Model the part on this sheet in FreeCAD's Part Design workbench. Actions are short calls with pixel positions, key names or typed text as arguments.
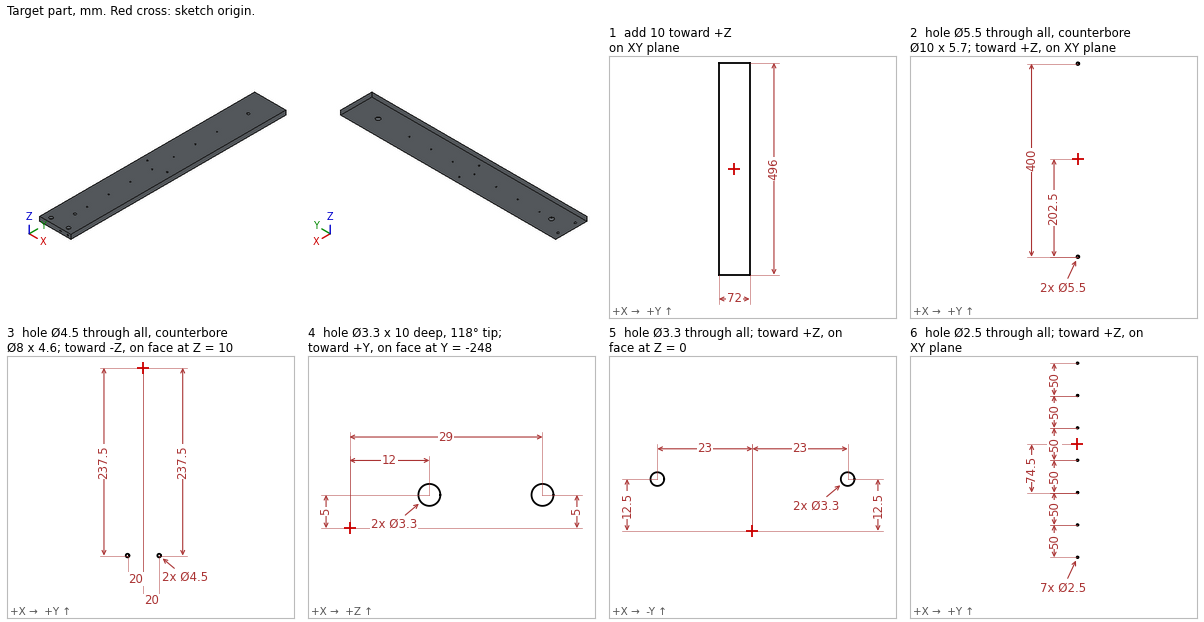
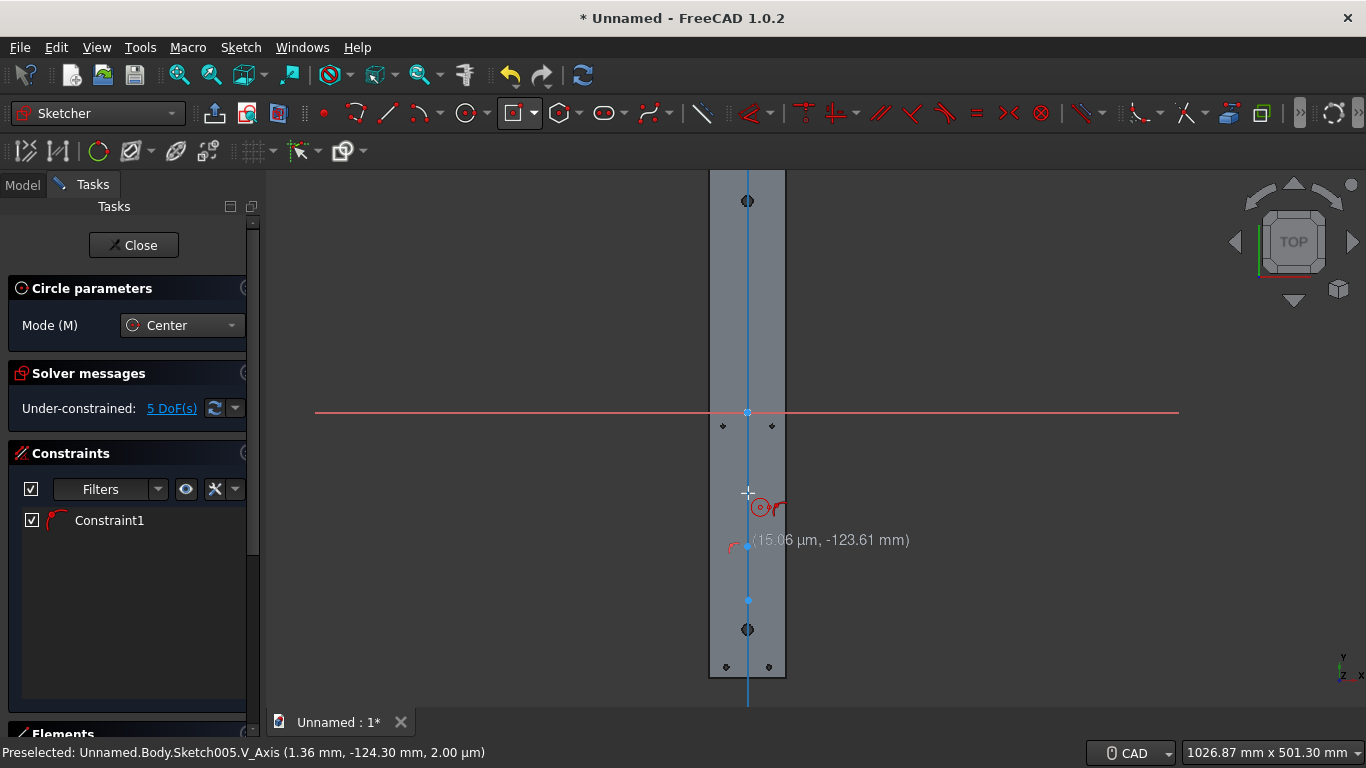
click(748, 493)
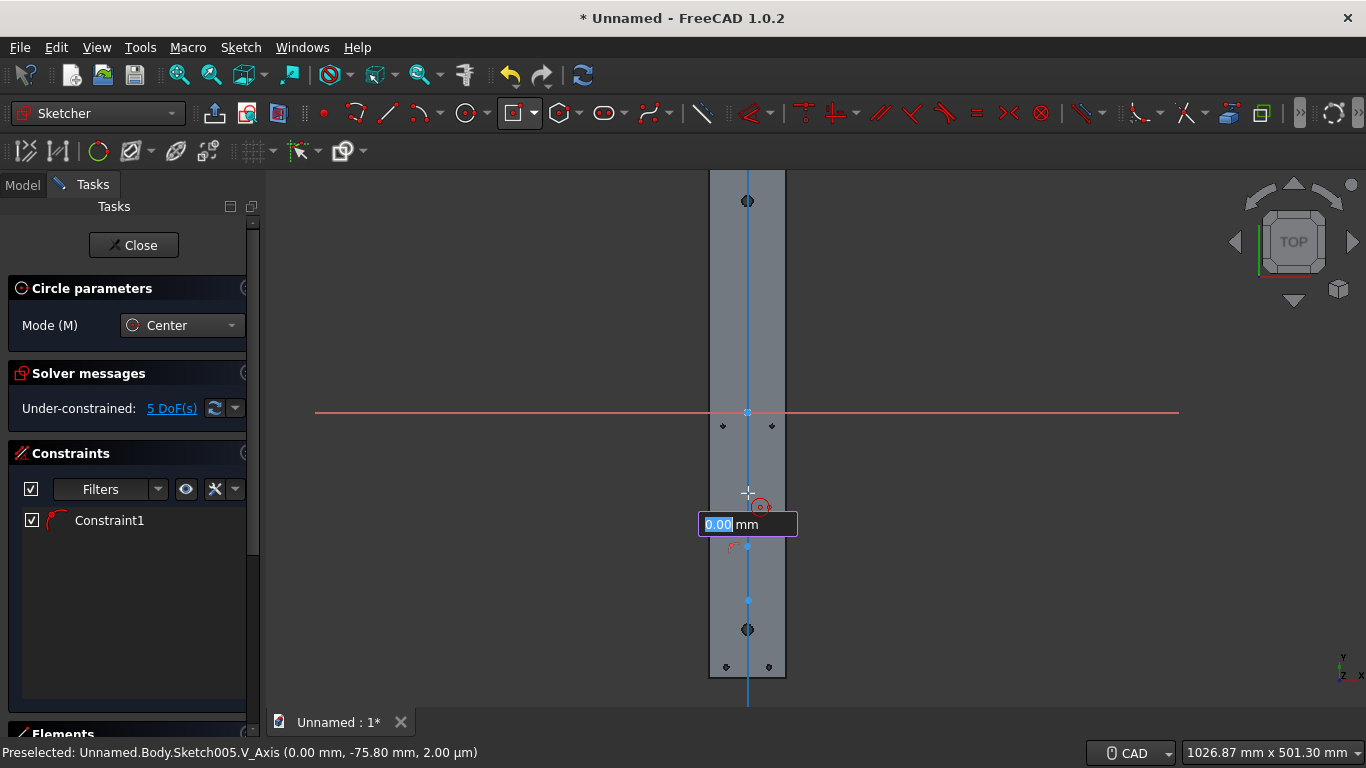
scroll(749, 492, up, 13)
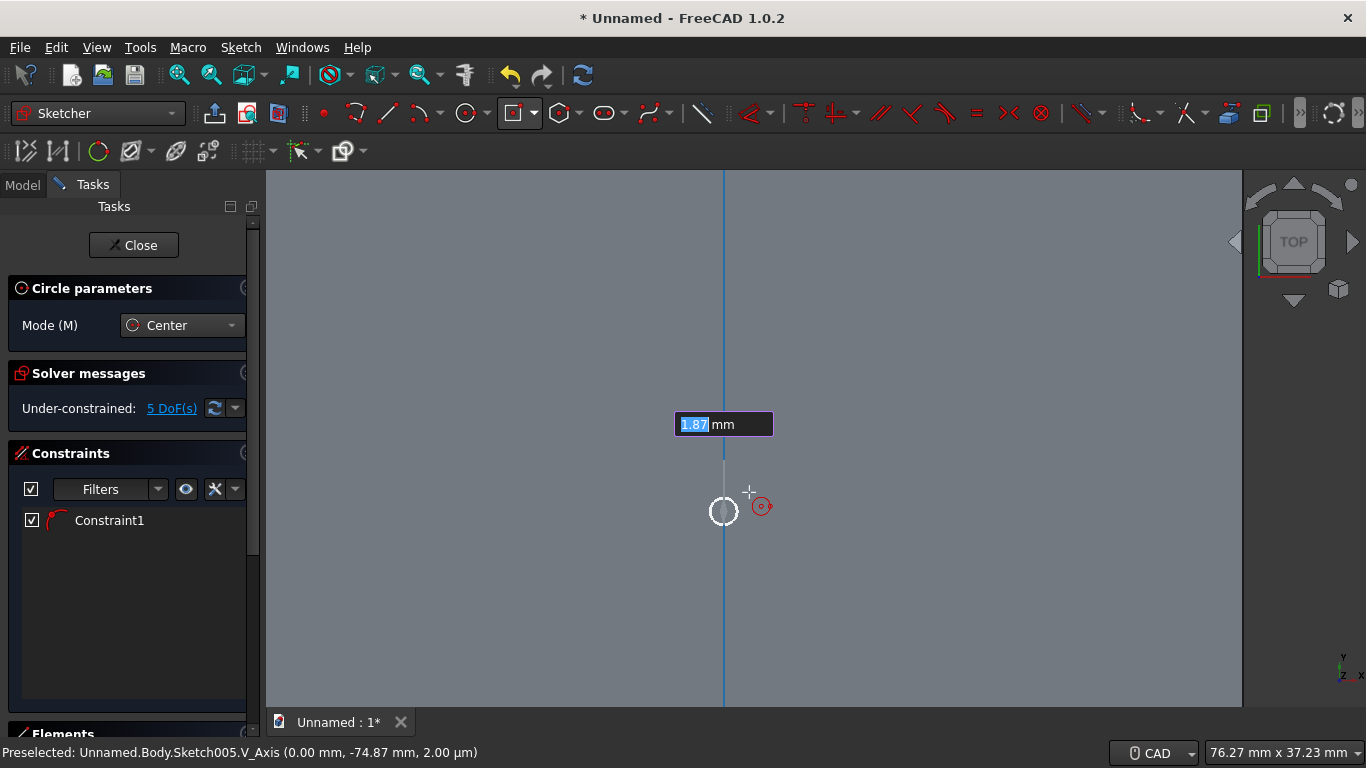
click(741, 486)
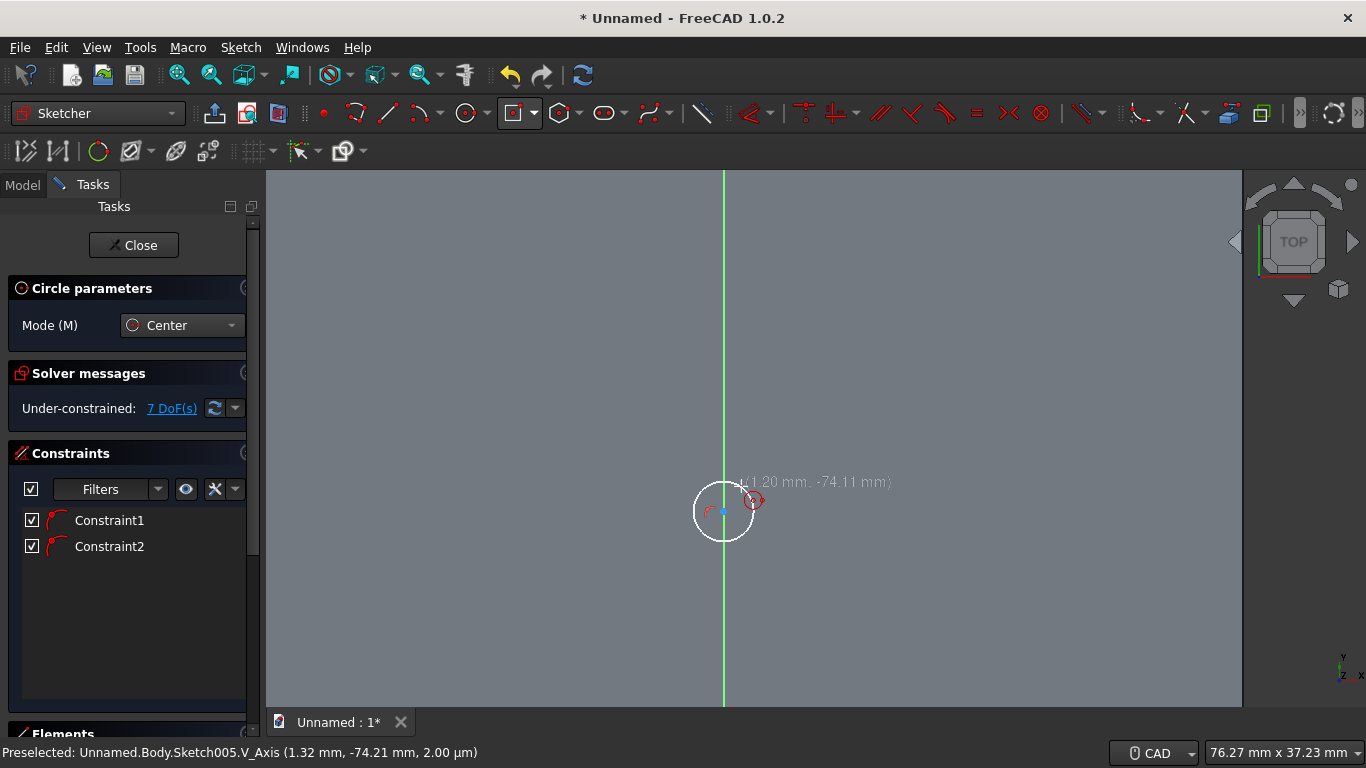
scroll(749, 492, down, 13)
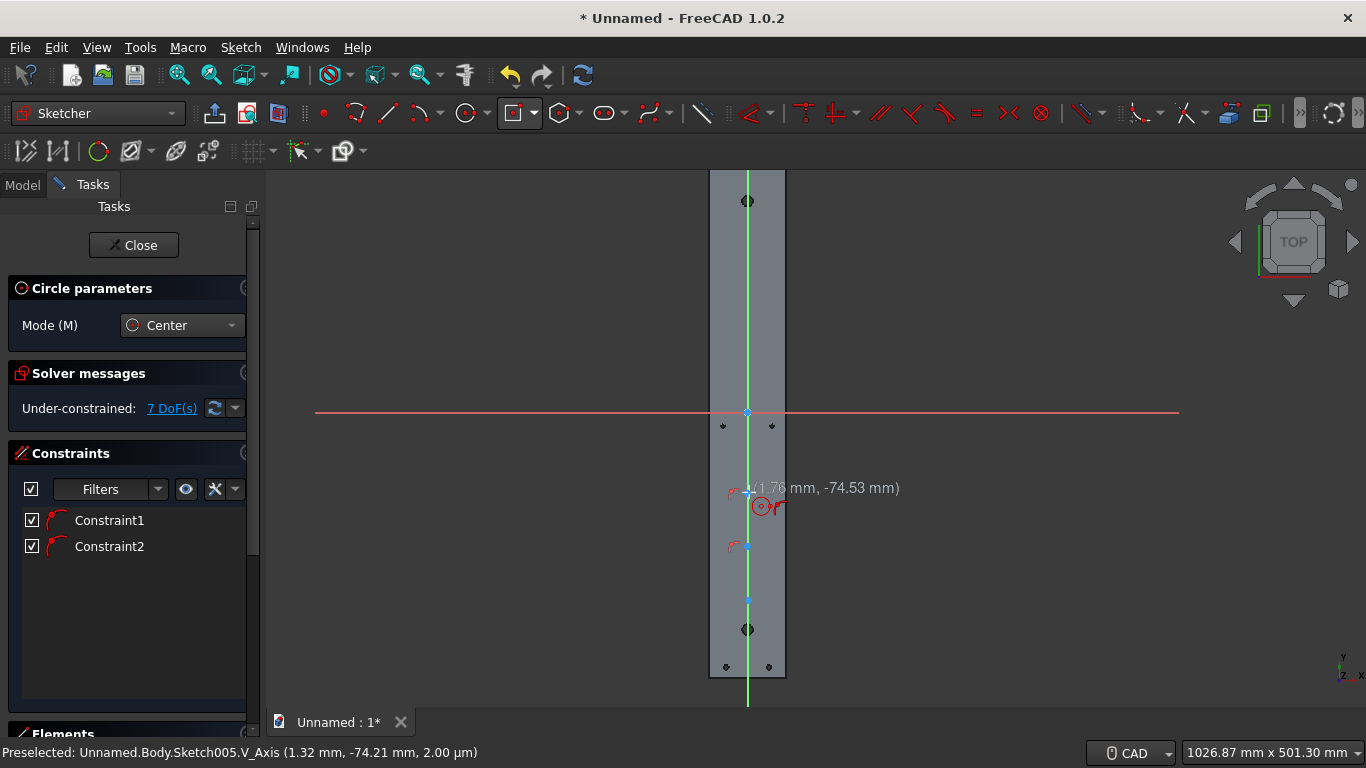
scroll(748, 439, up, 15)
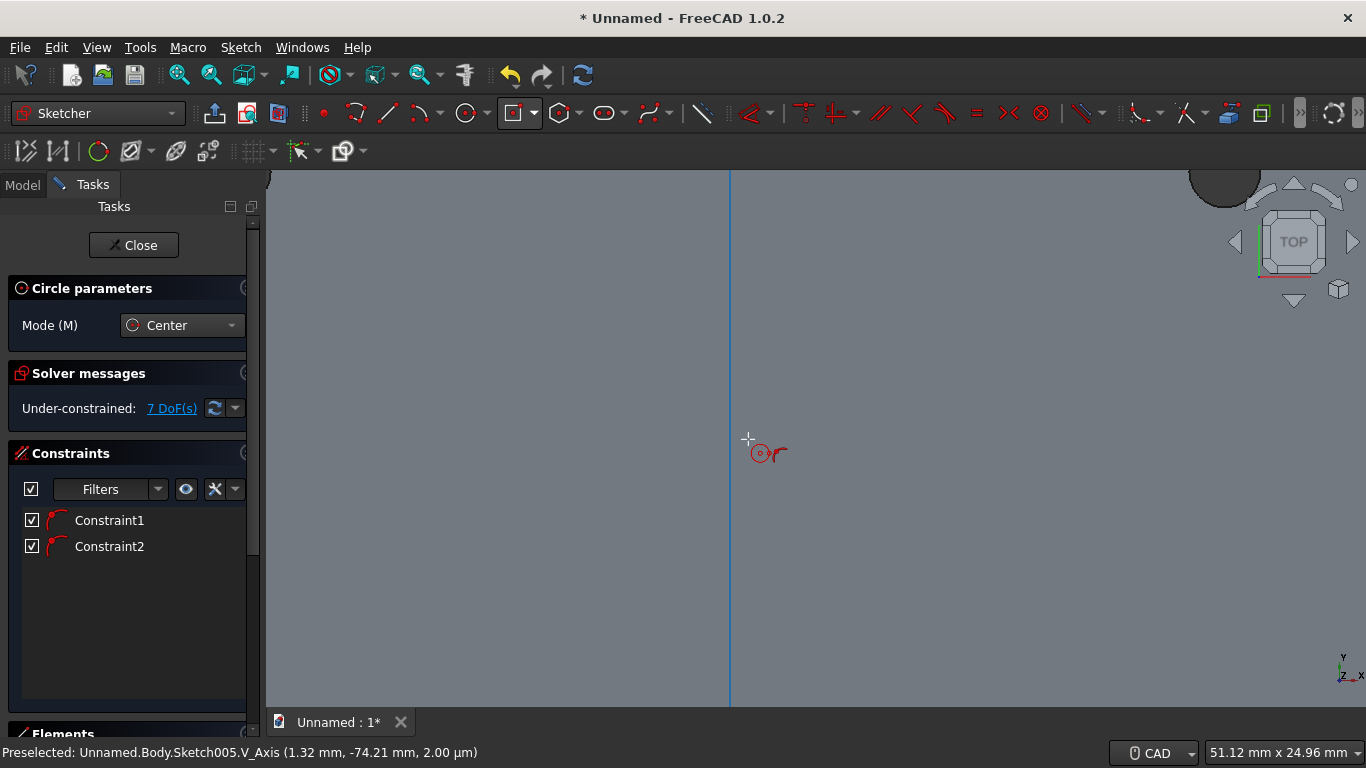
scroll(748, 439, down, 15)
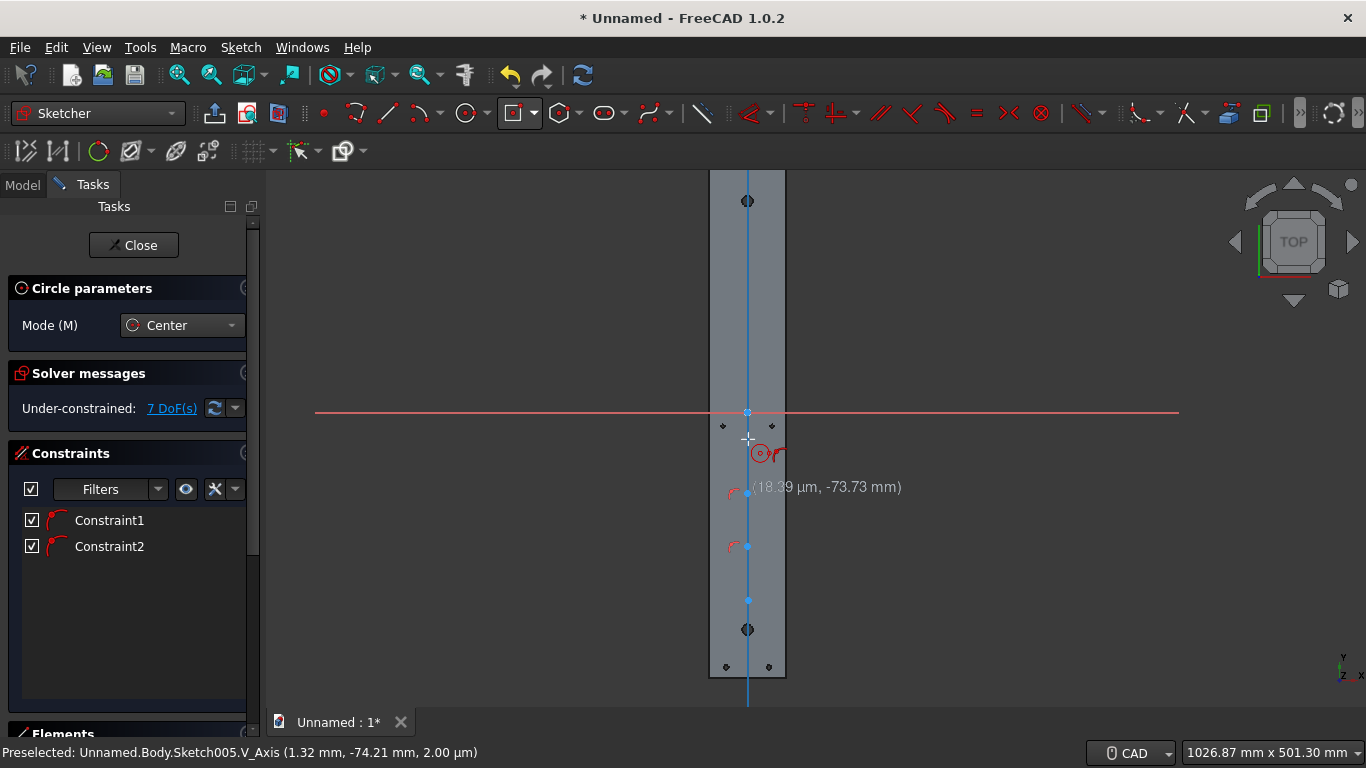
click(748, 439)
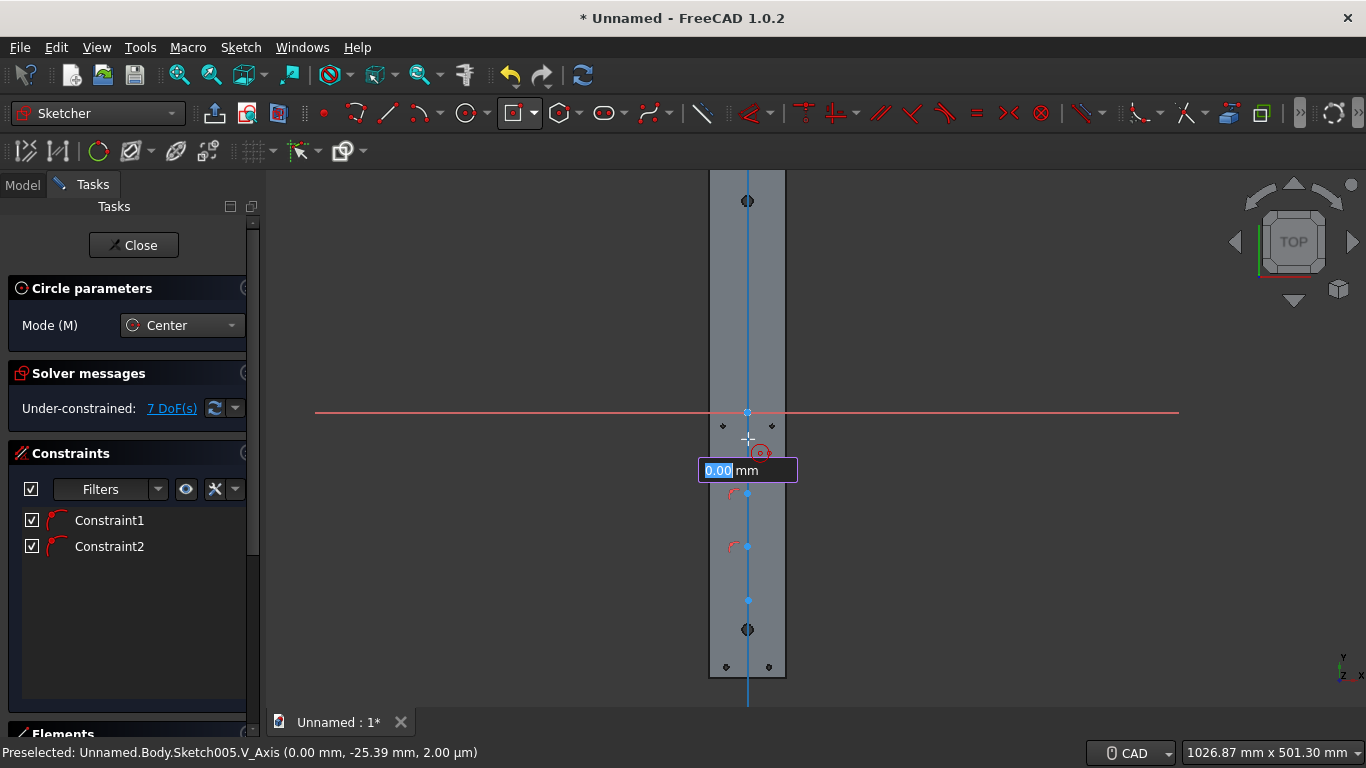
scroll(749, 439, up, 13)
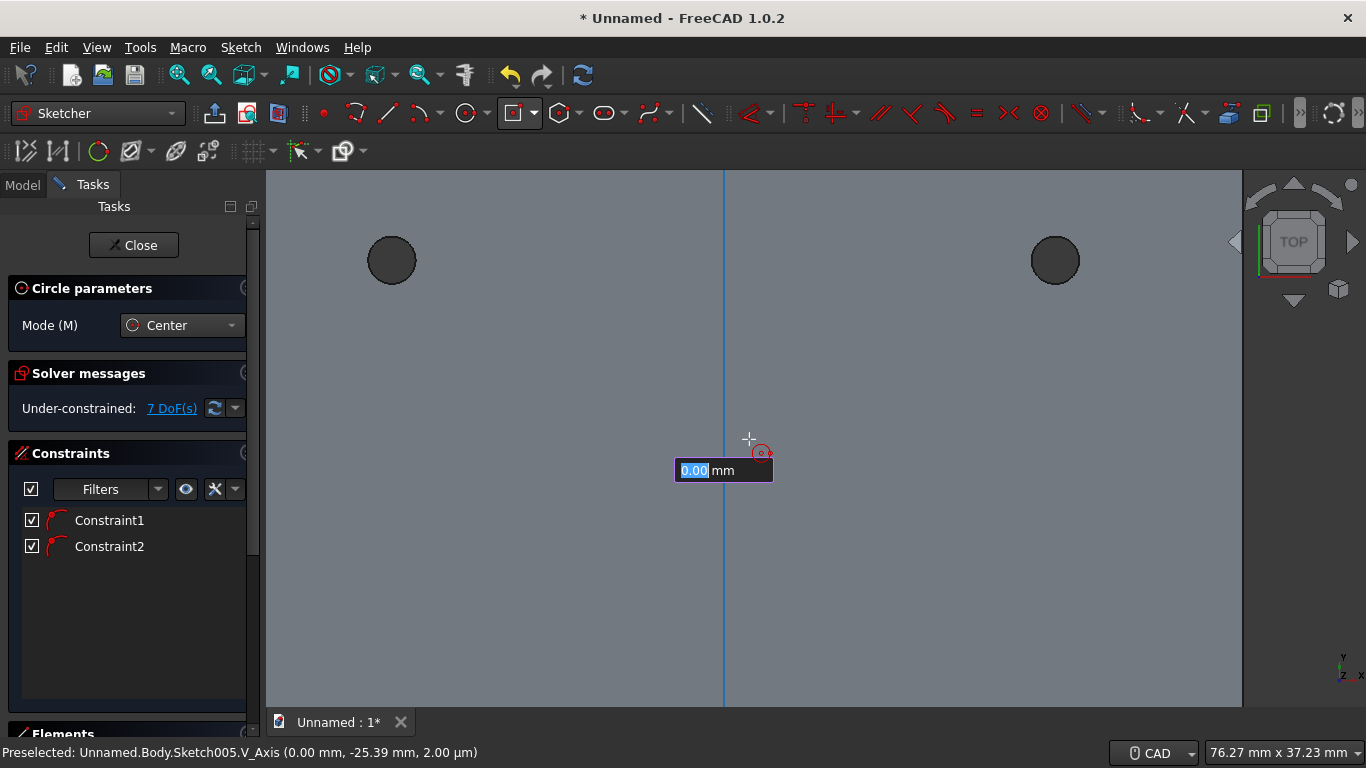
click(741, 427)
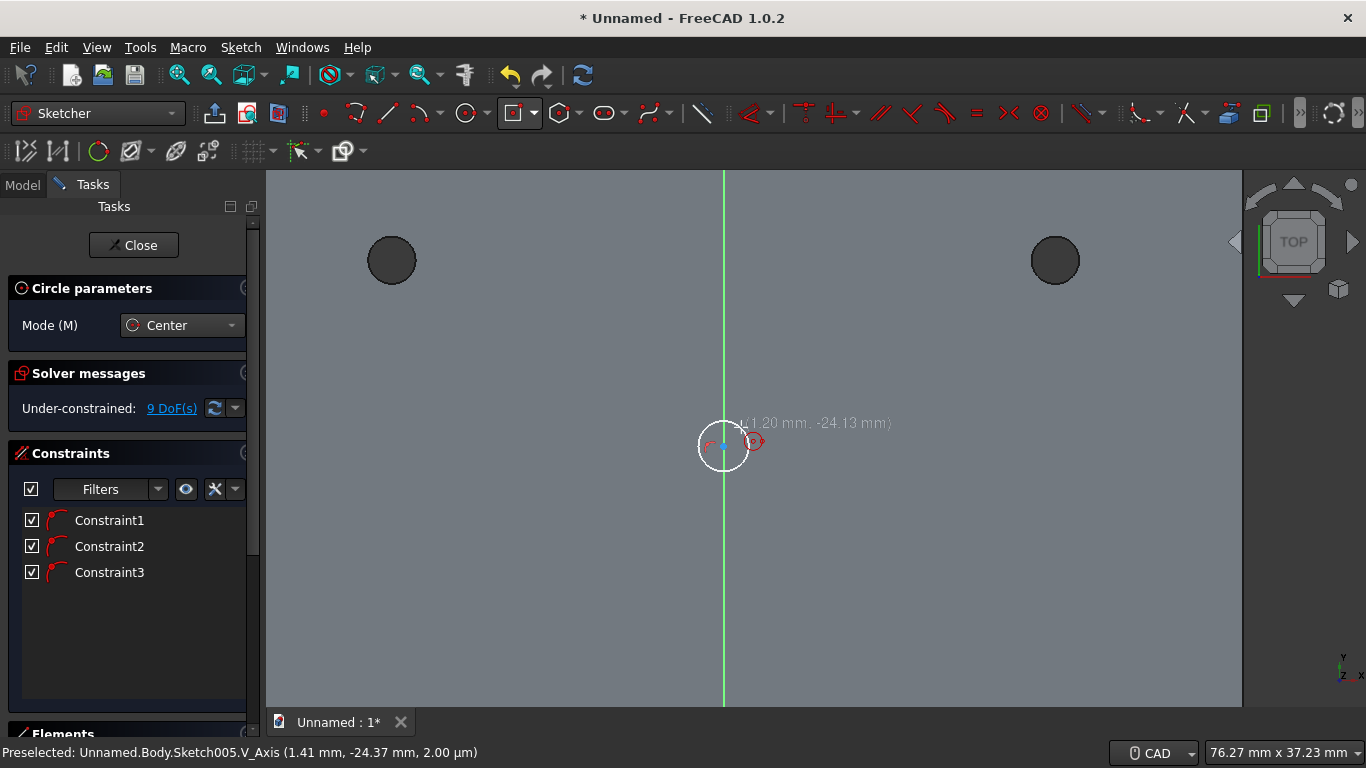
scroll(749, 439, down, 13)